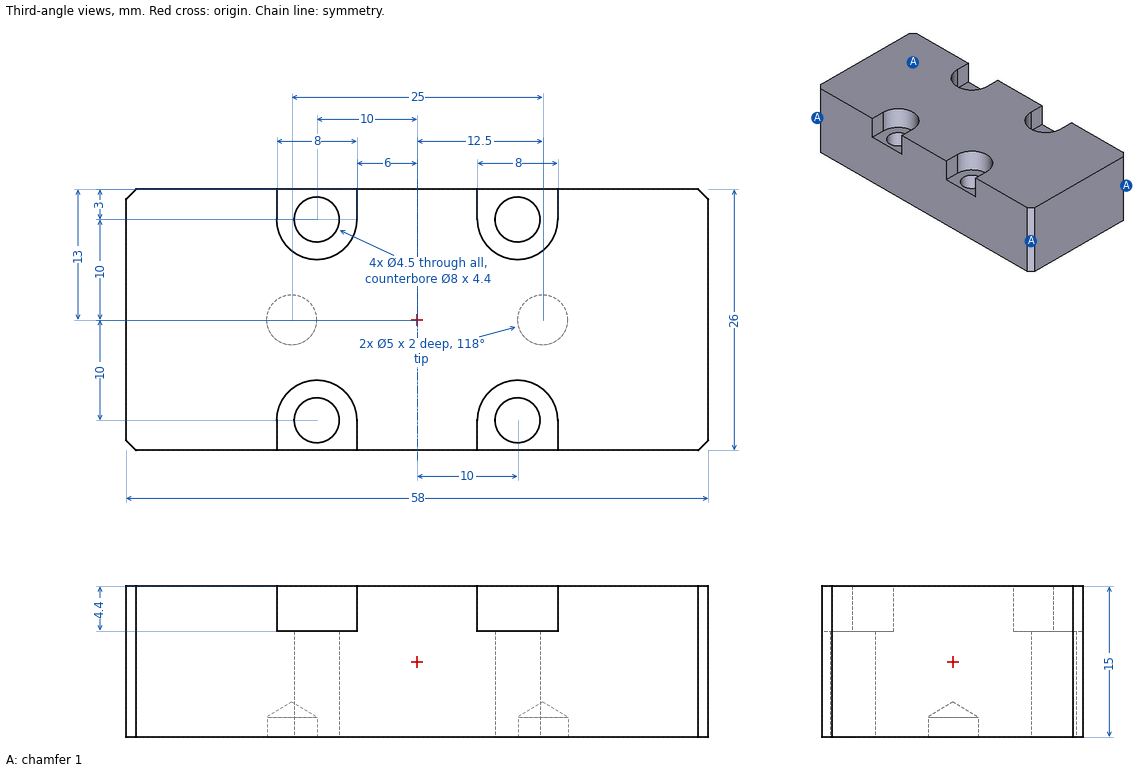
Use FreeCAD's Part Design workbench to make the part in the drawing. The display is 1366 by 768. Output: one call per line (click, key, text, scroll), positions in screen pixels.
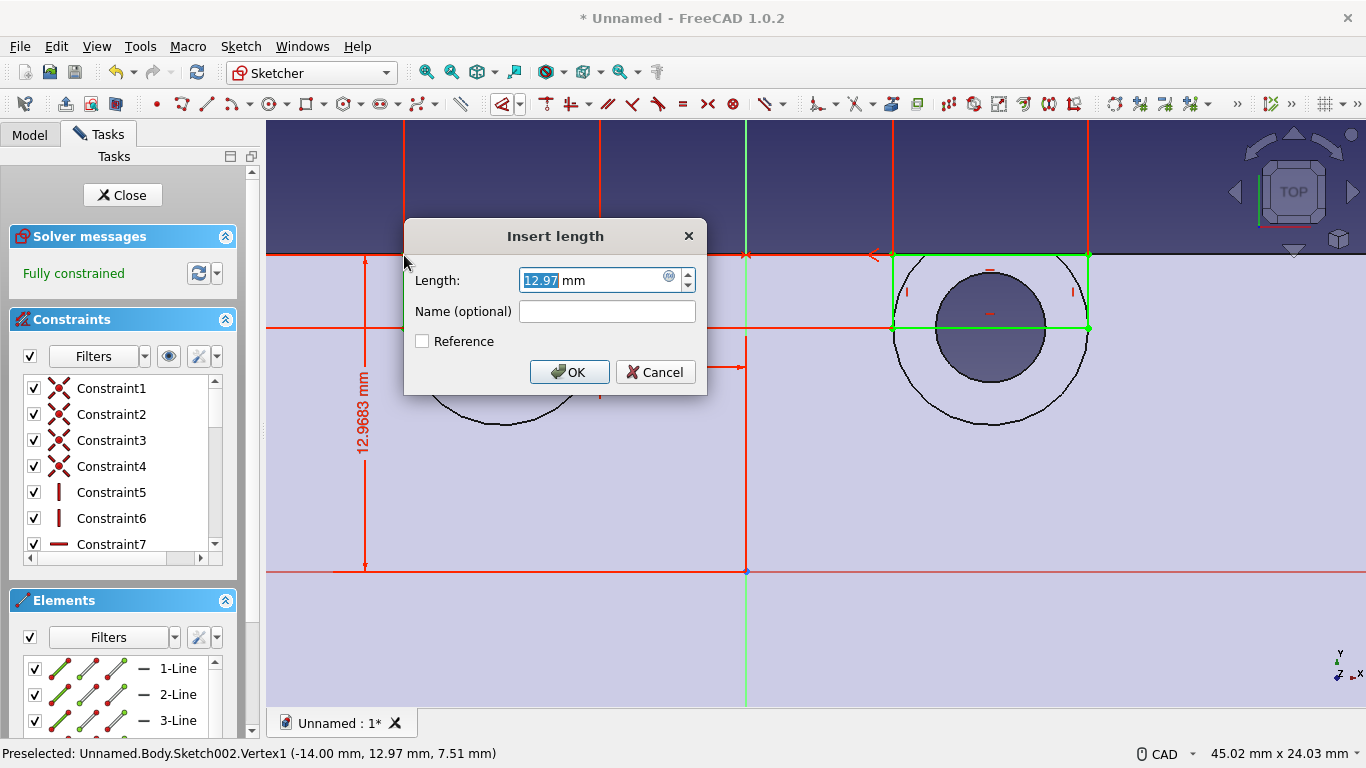
text(13)
key(Return)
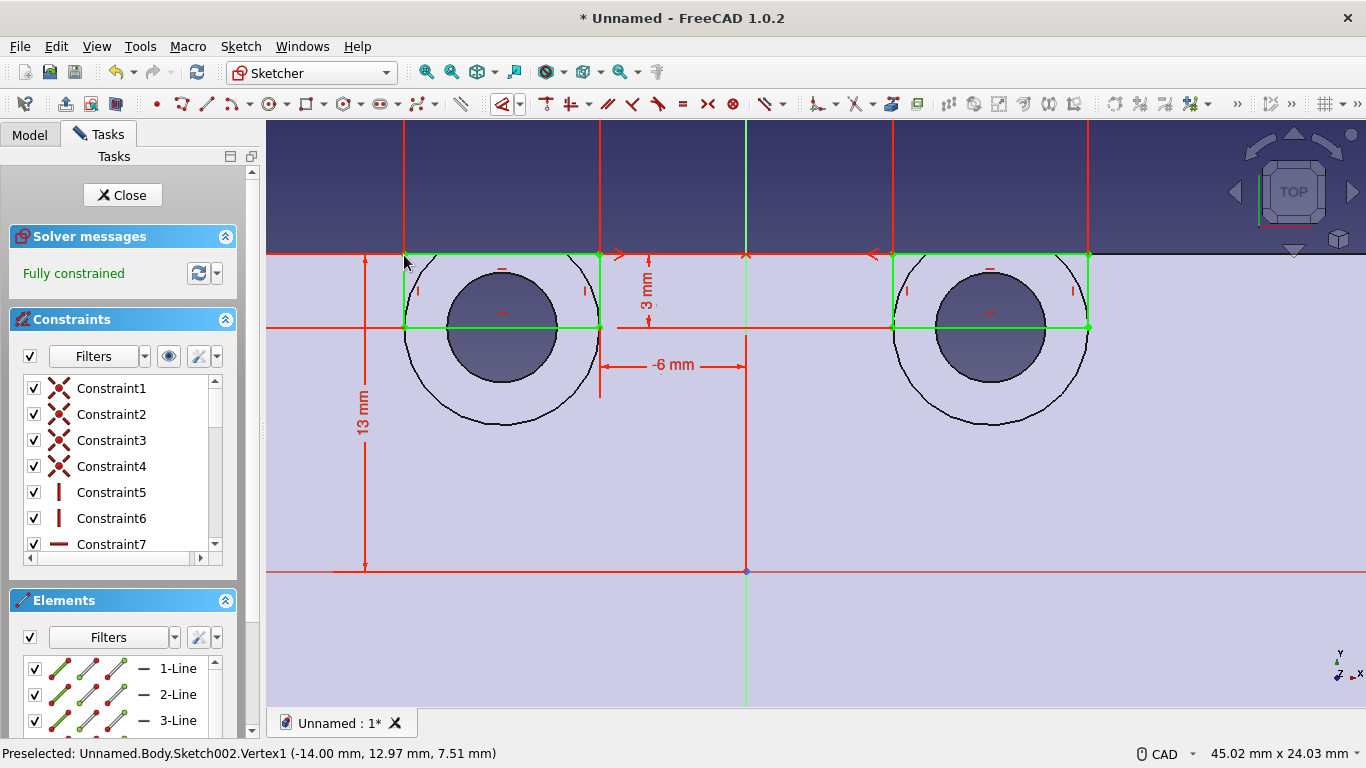
click(123, 195)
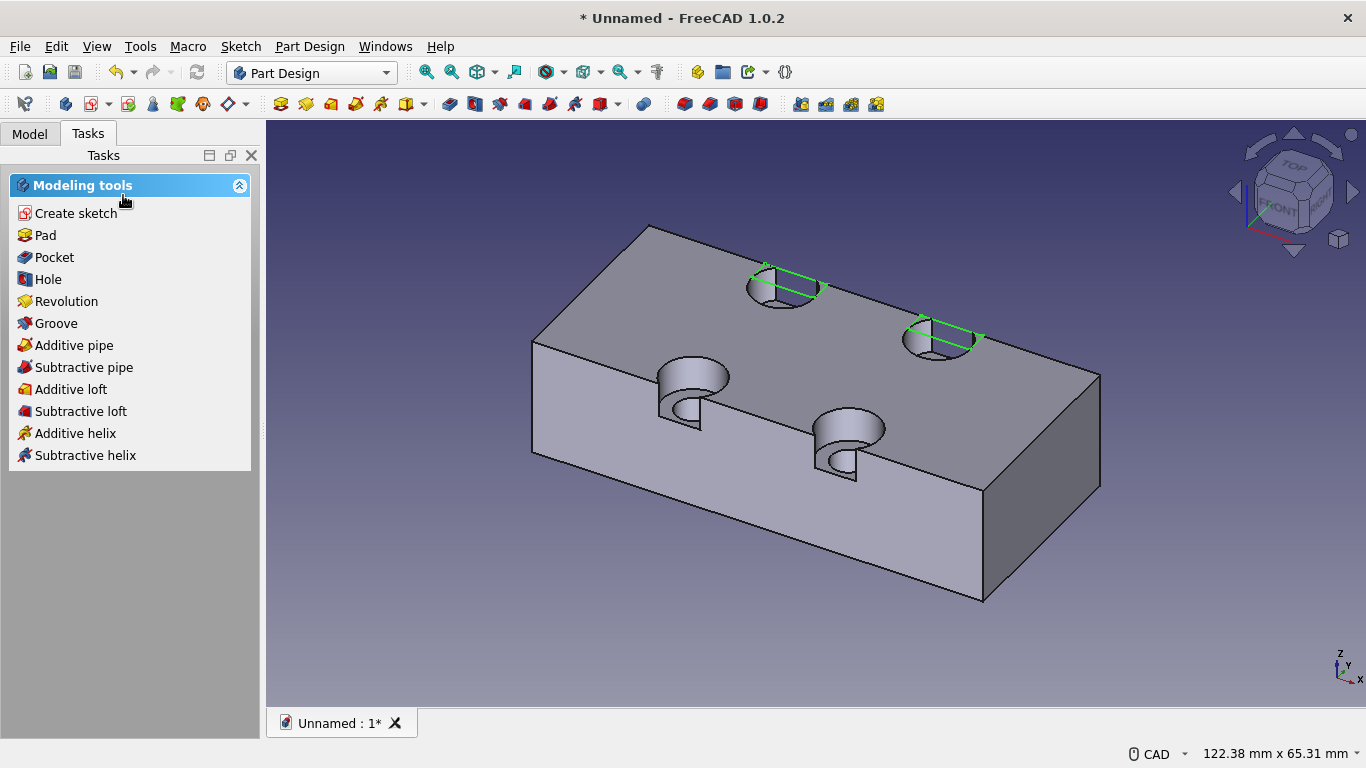
click(450, 104)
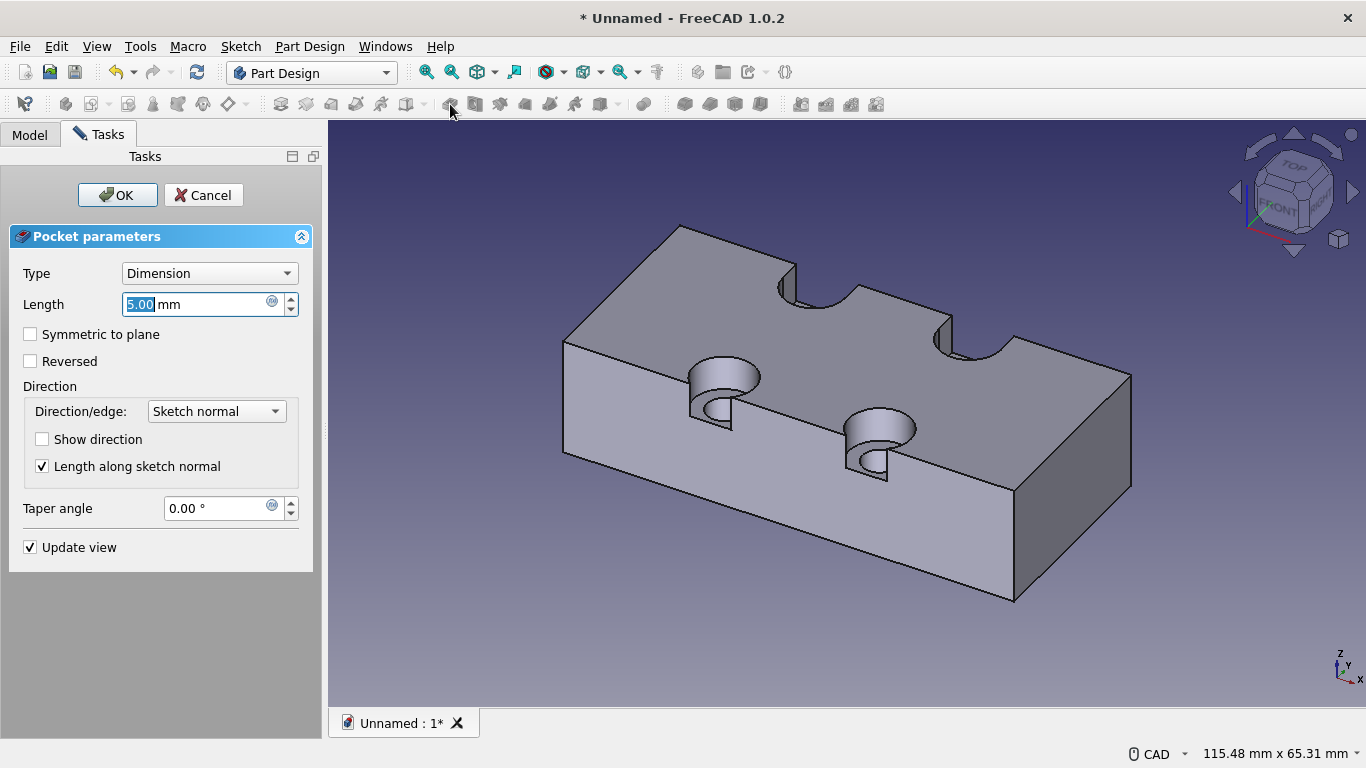
text(4.4)
key(Tab)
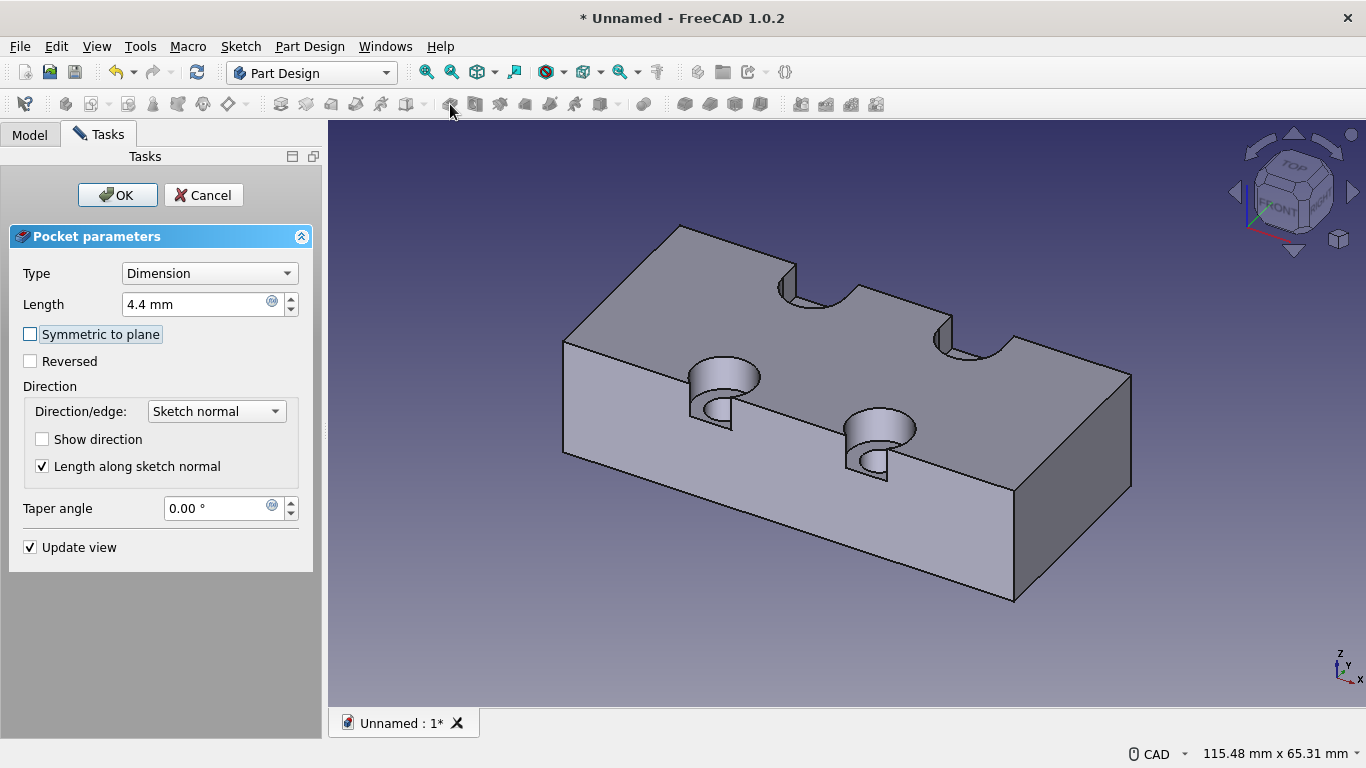
click(118, 195)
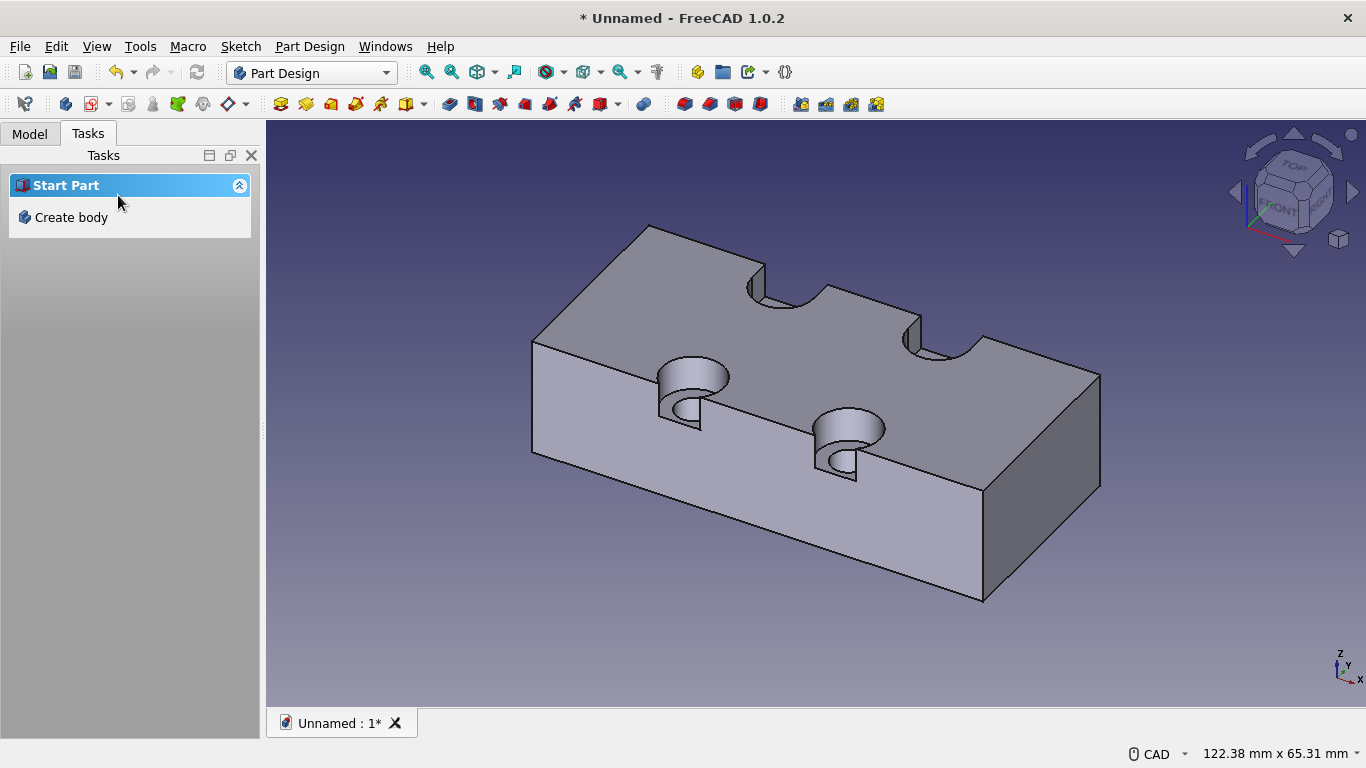
click(30, 134)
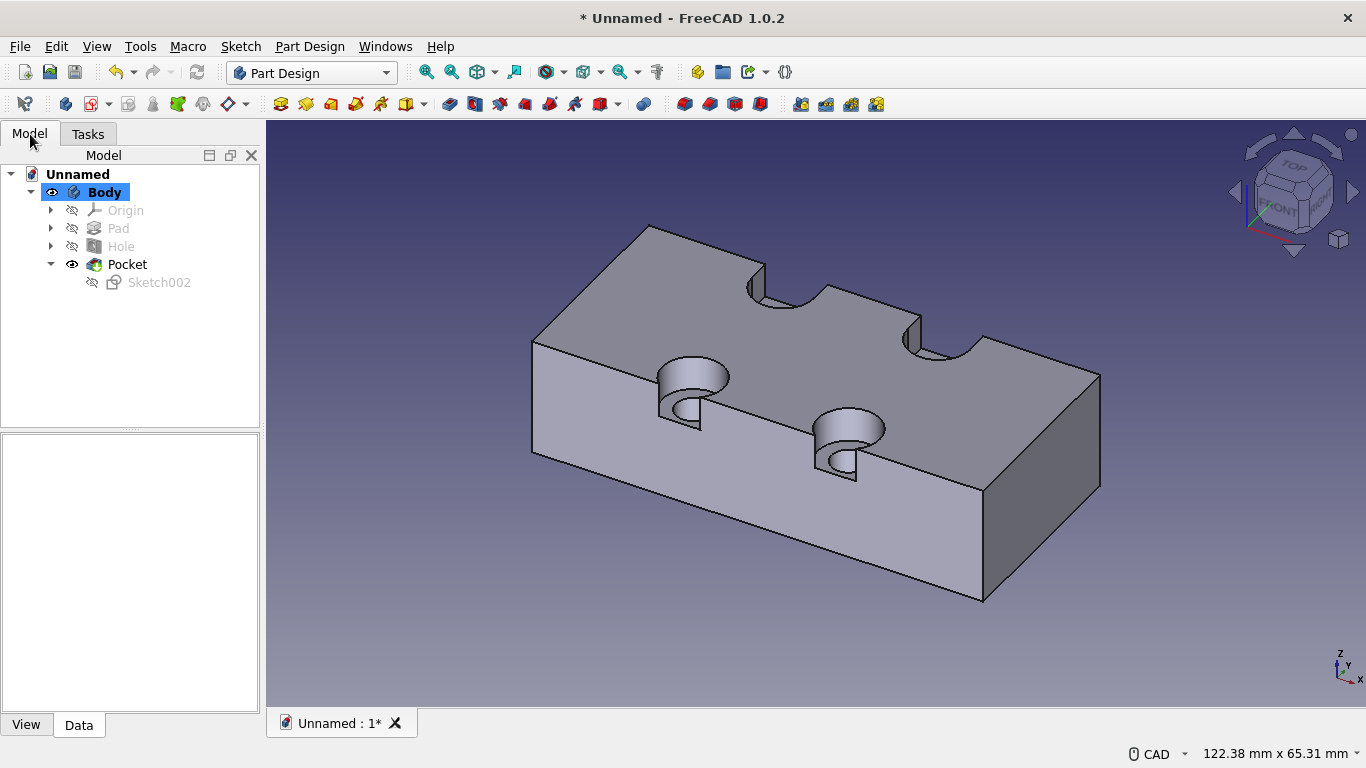
click(117, 264)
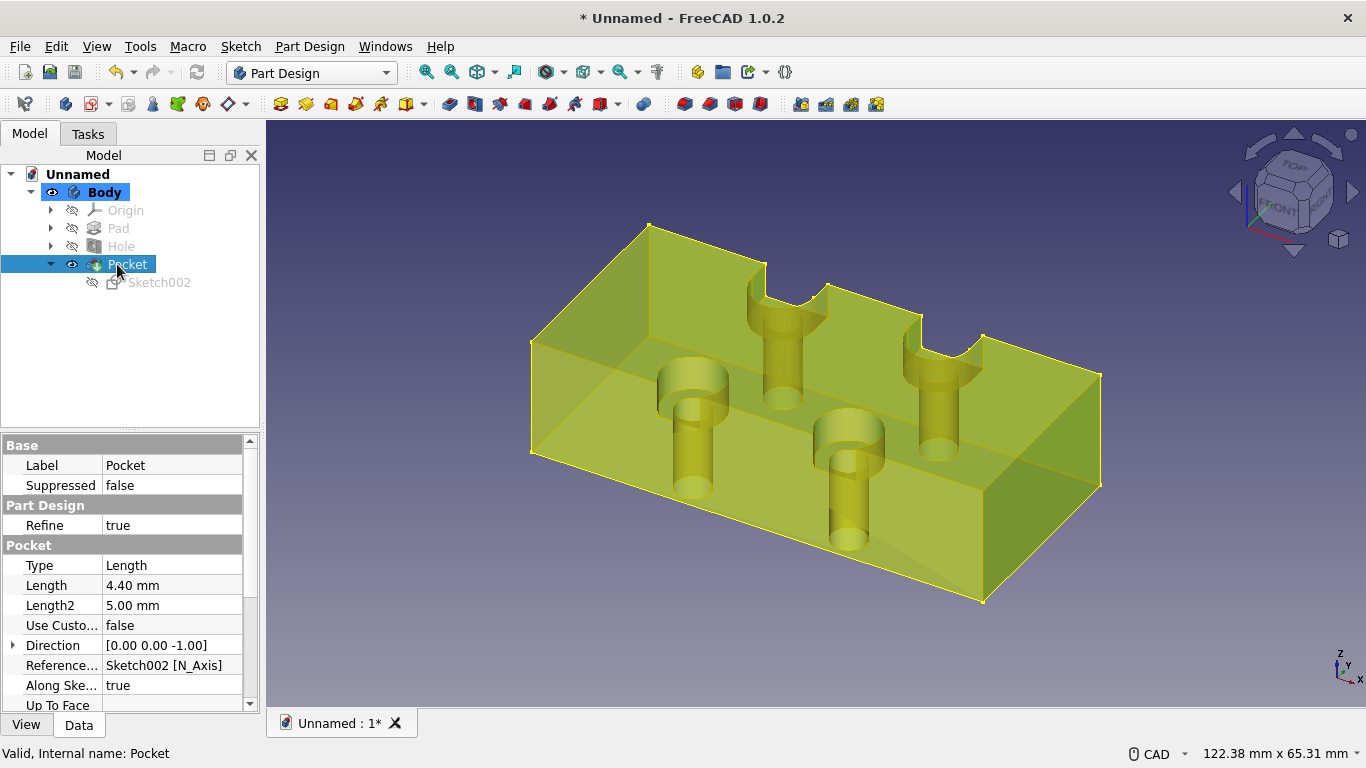
click(801, 104)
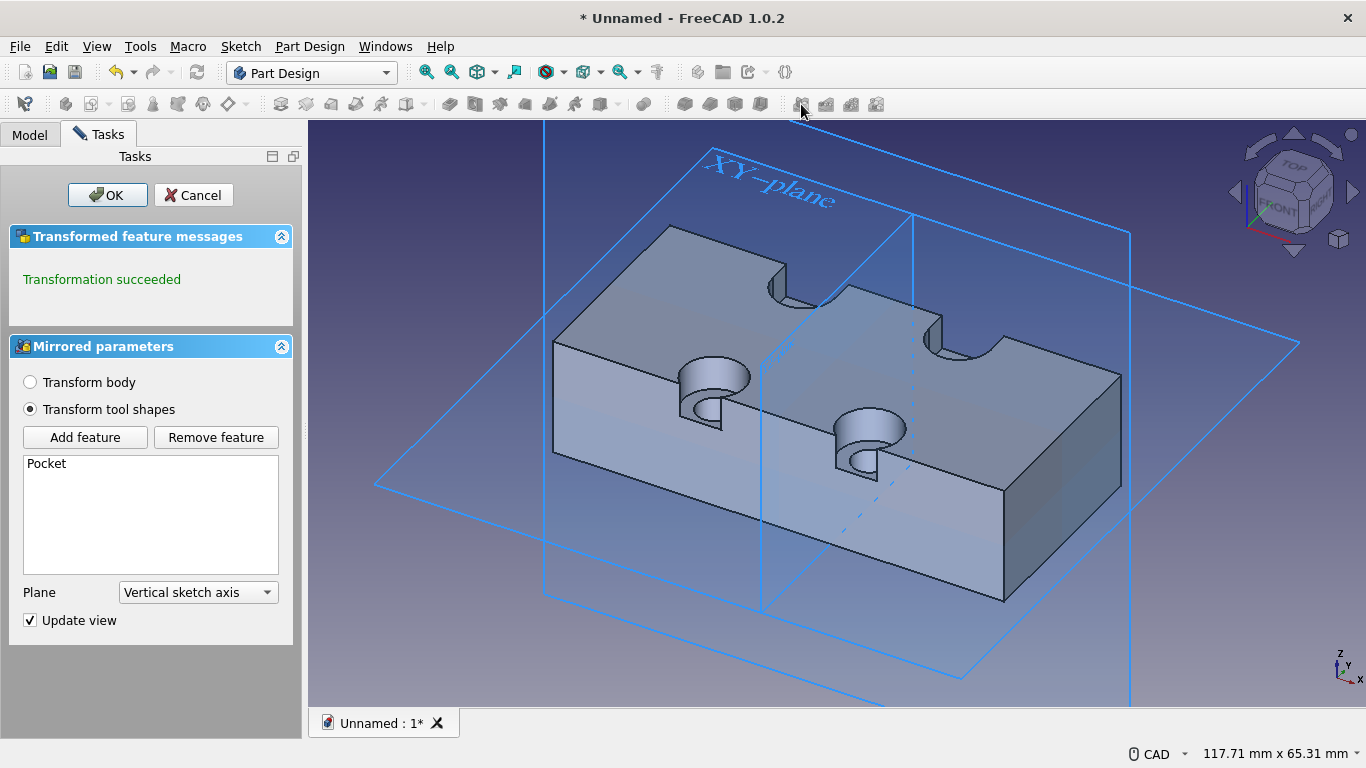
click(199, 592)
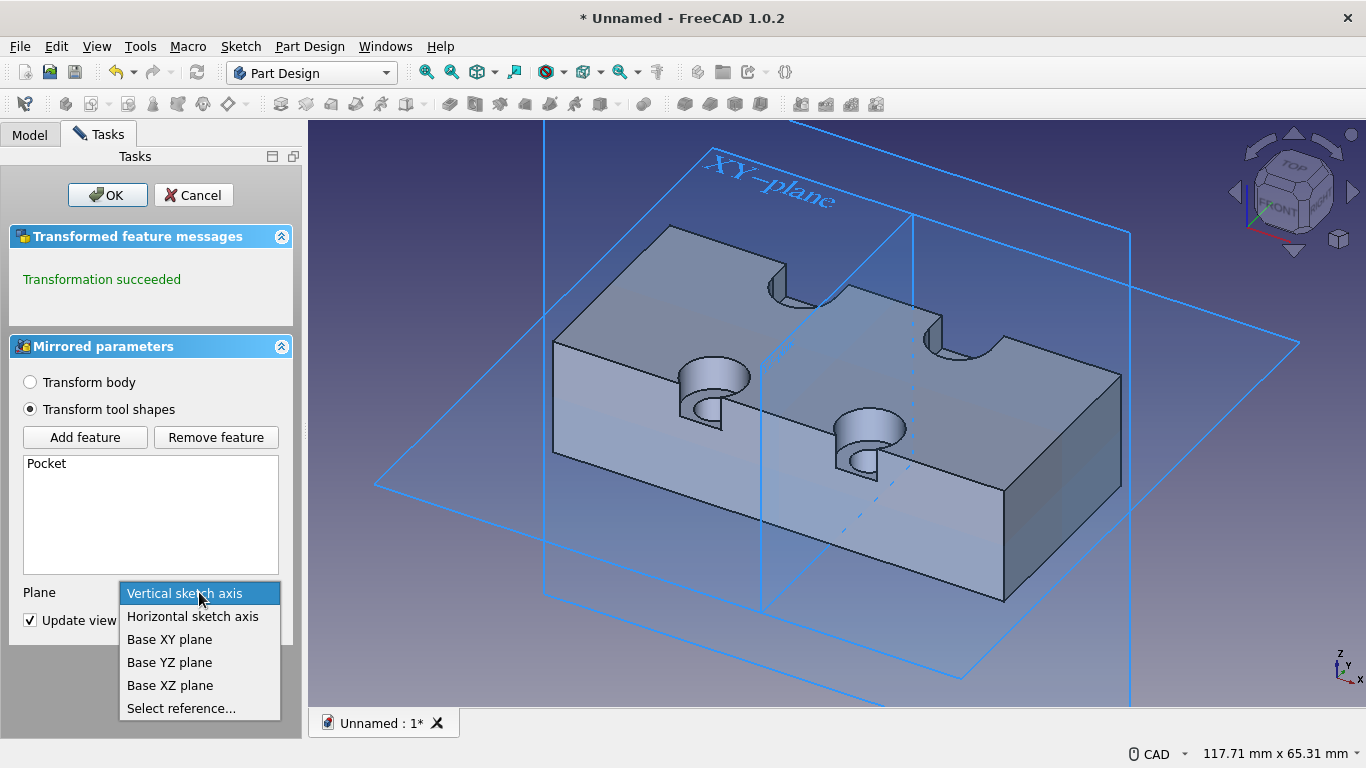
click(198, 686)